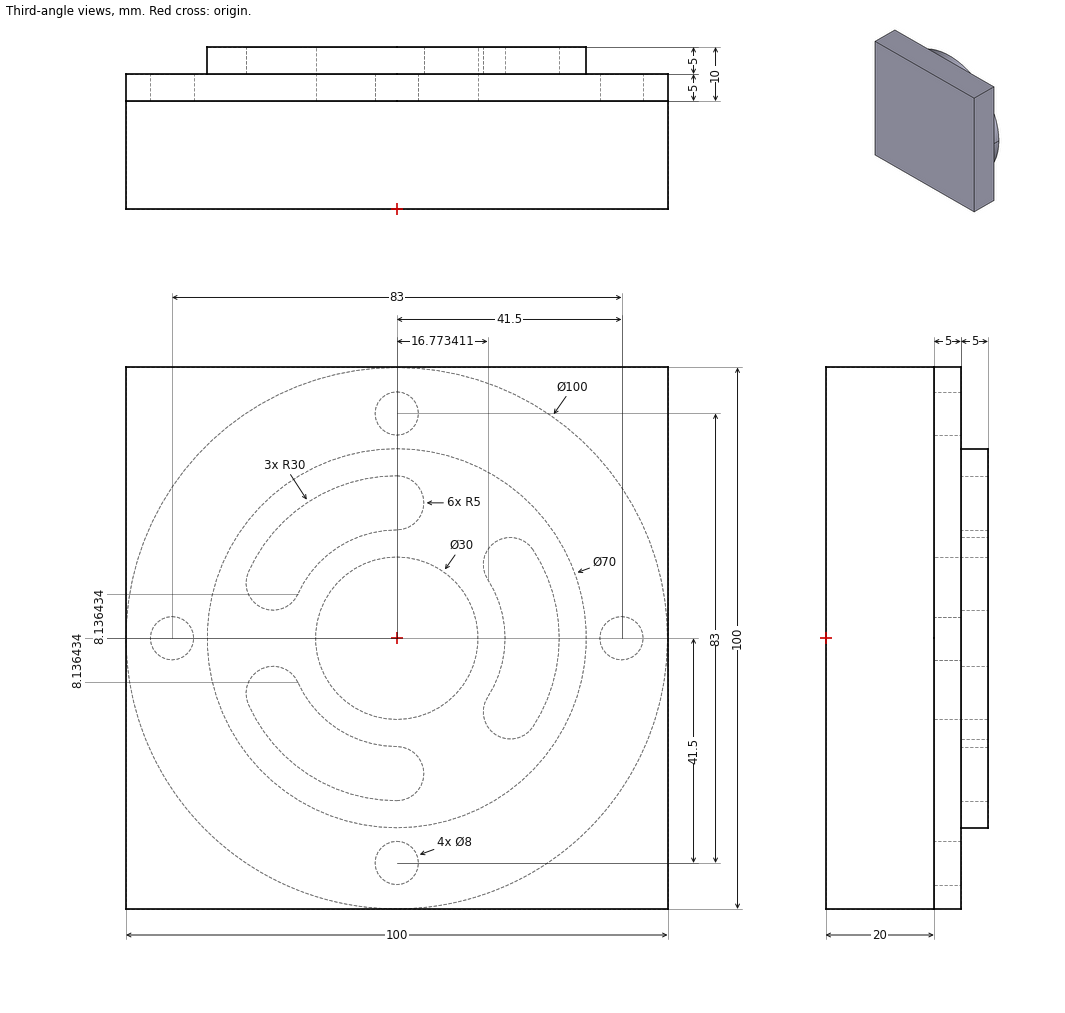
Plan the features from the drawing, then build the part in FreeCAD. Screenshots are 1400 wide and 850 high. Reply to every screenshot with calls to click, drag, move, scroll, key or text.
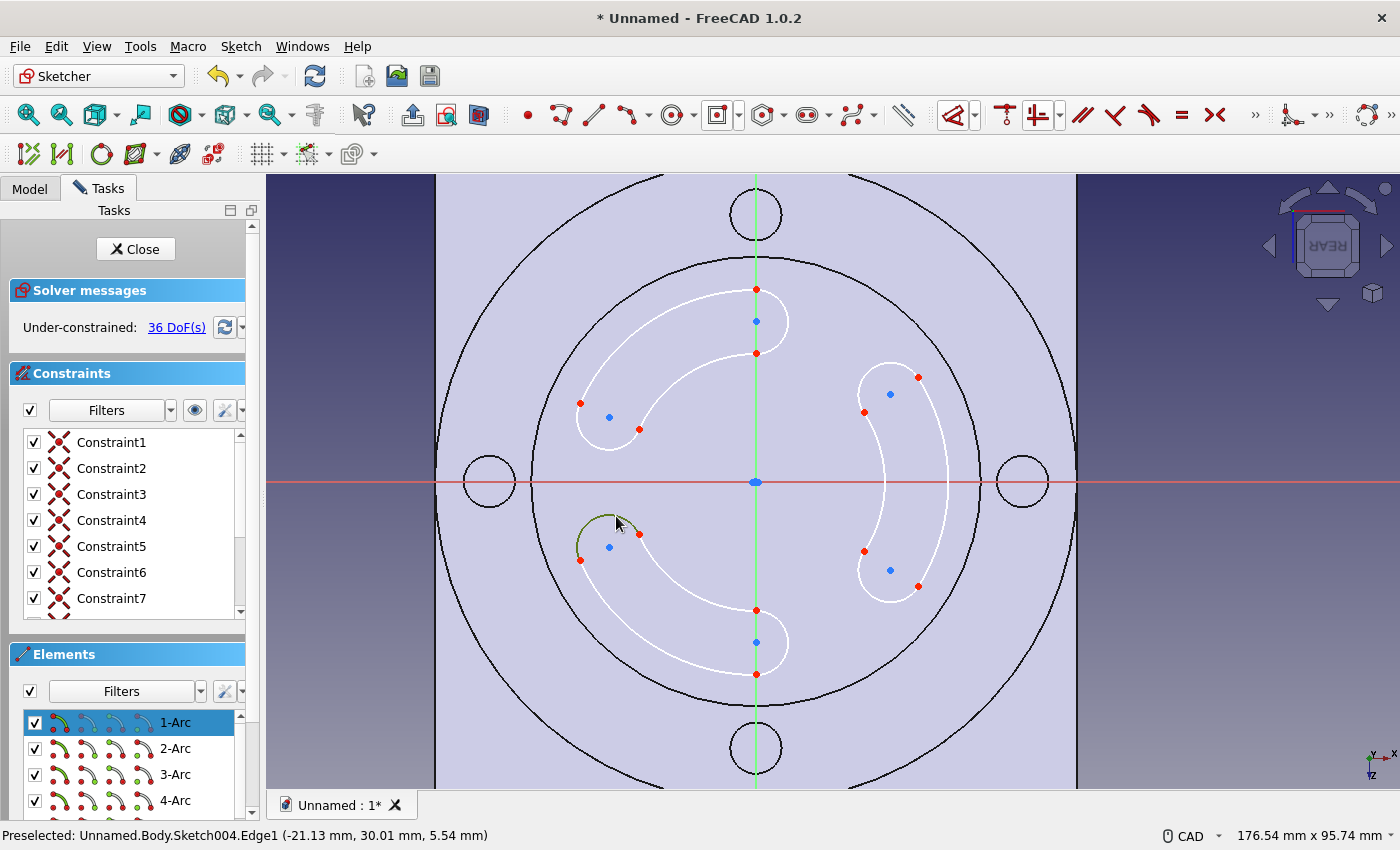
click(617, 616)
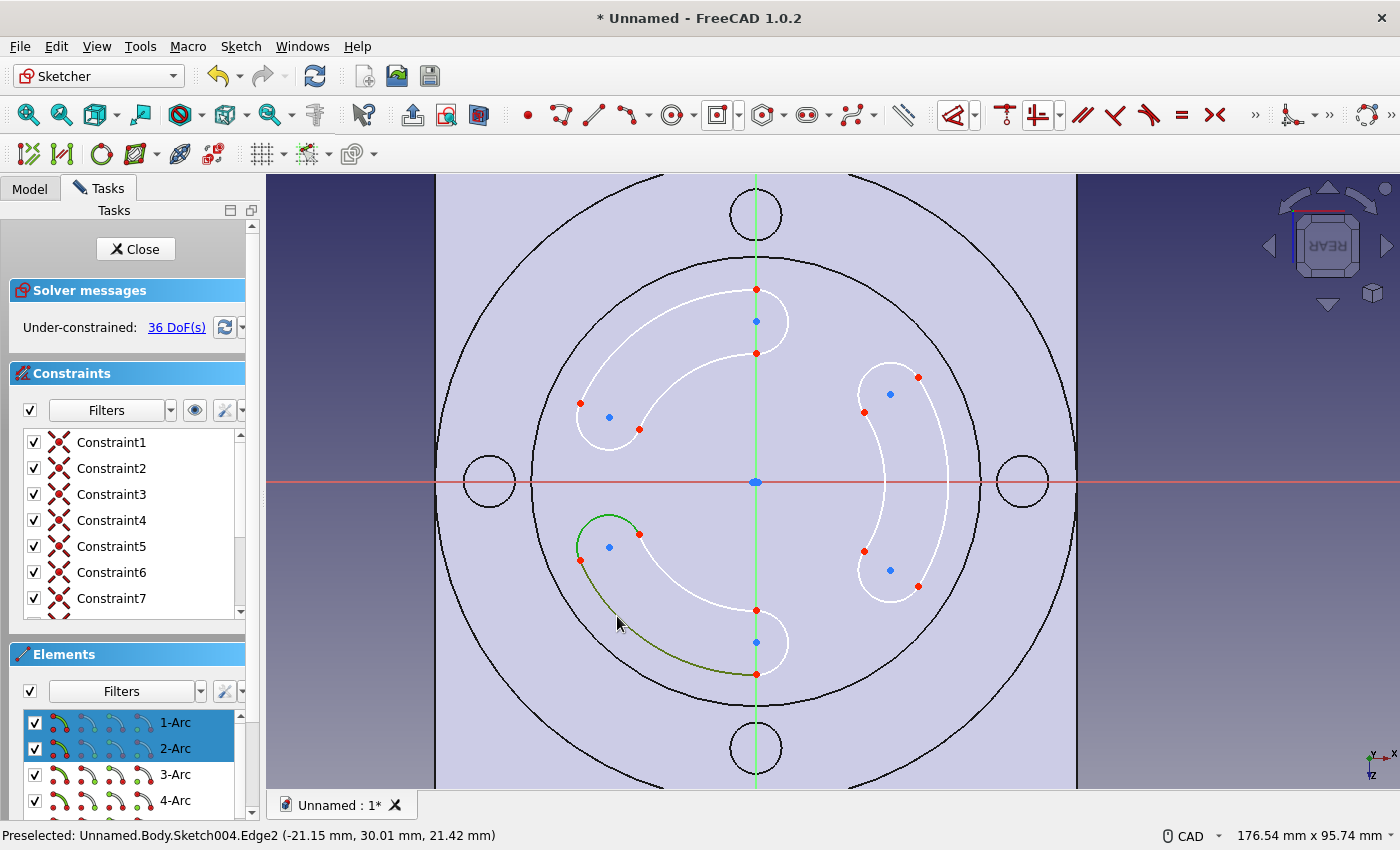
click(1149, 116)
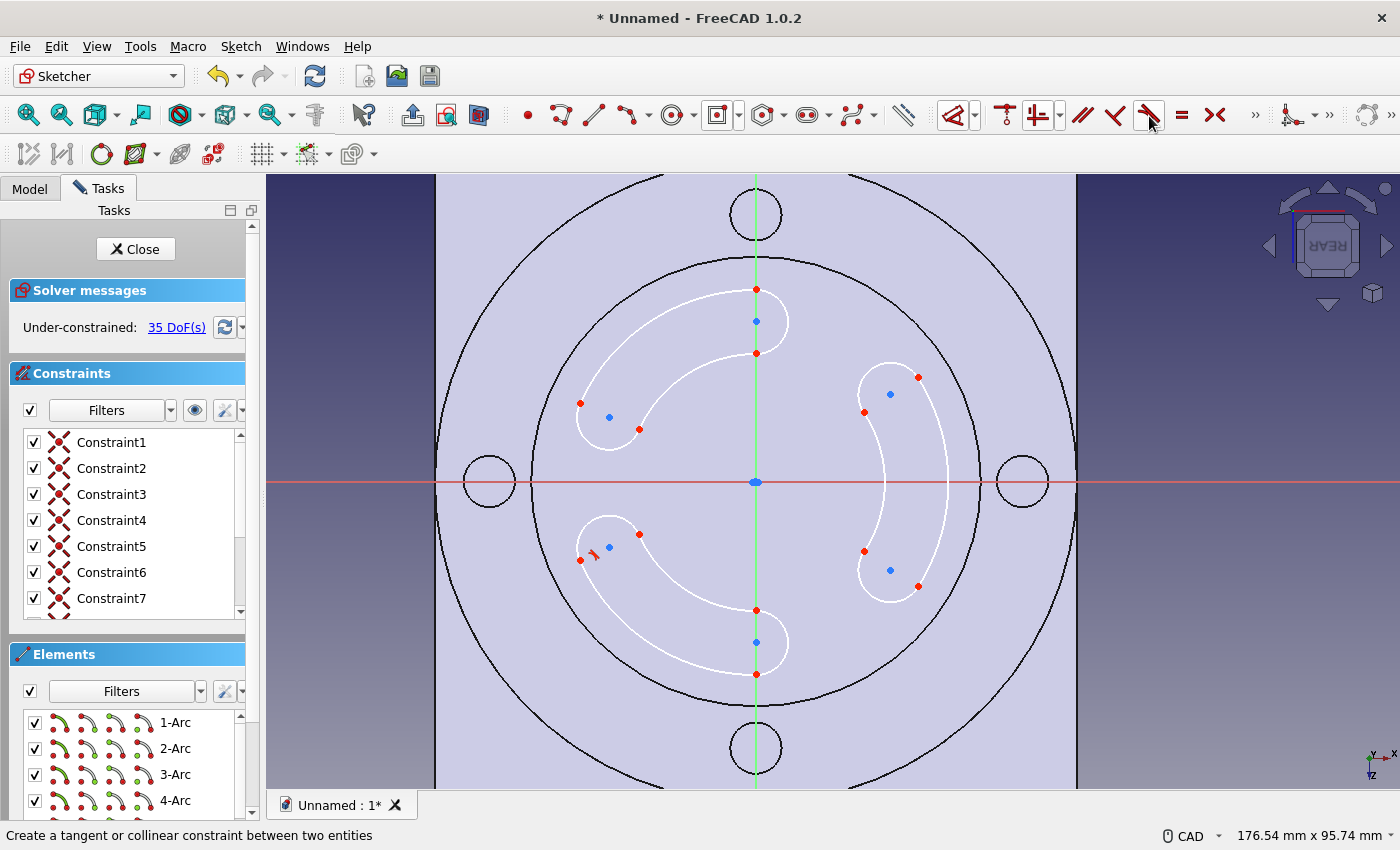
click(616, 516)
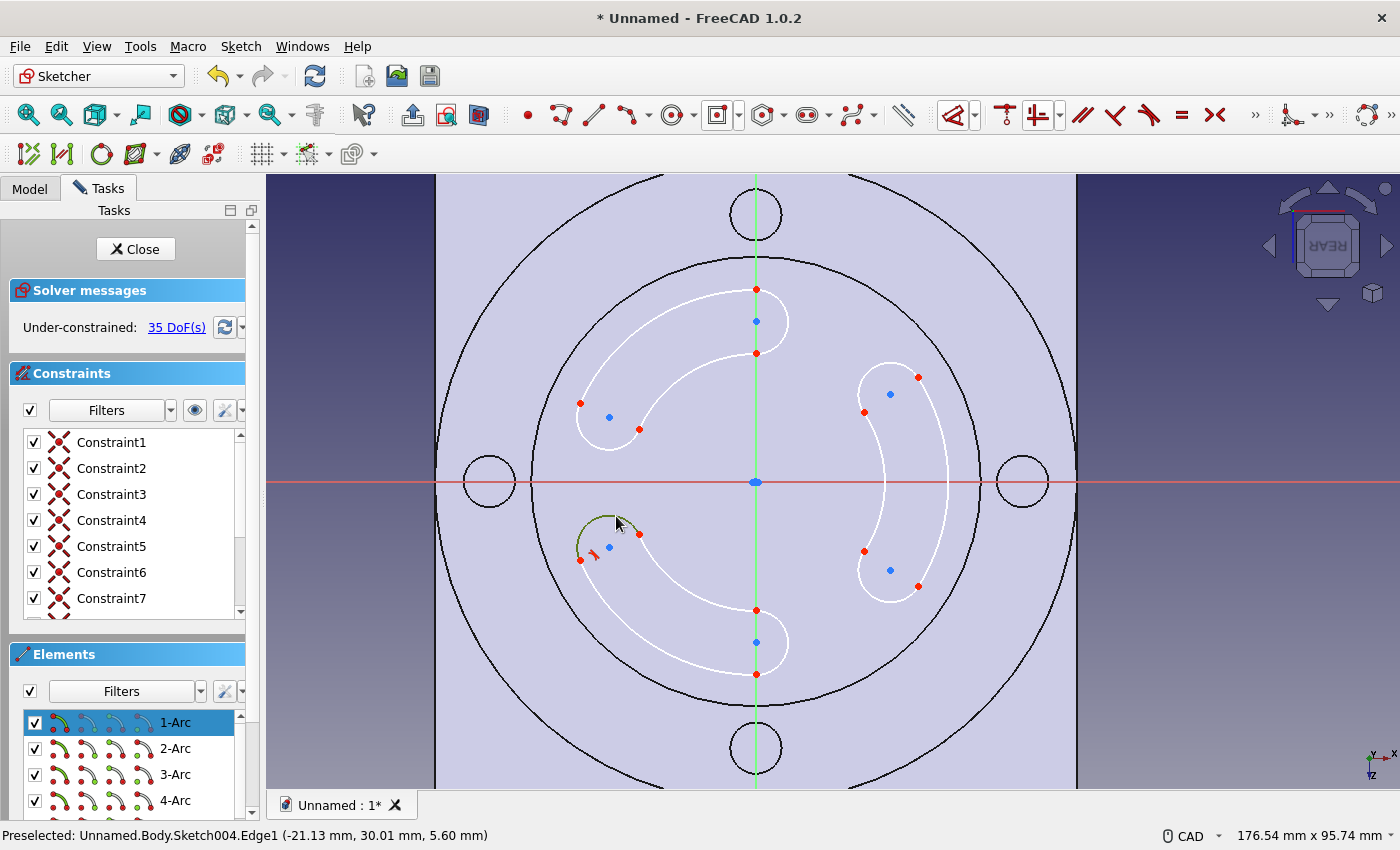
click(664, 571)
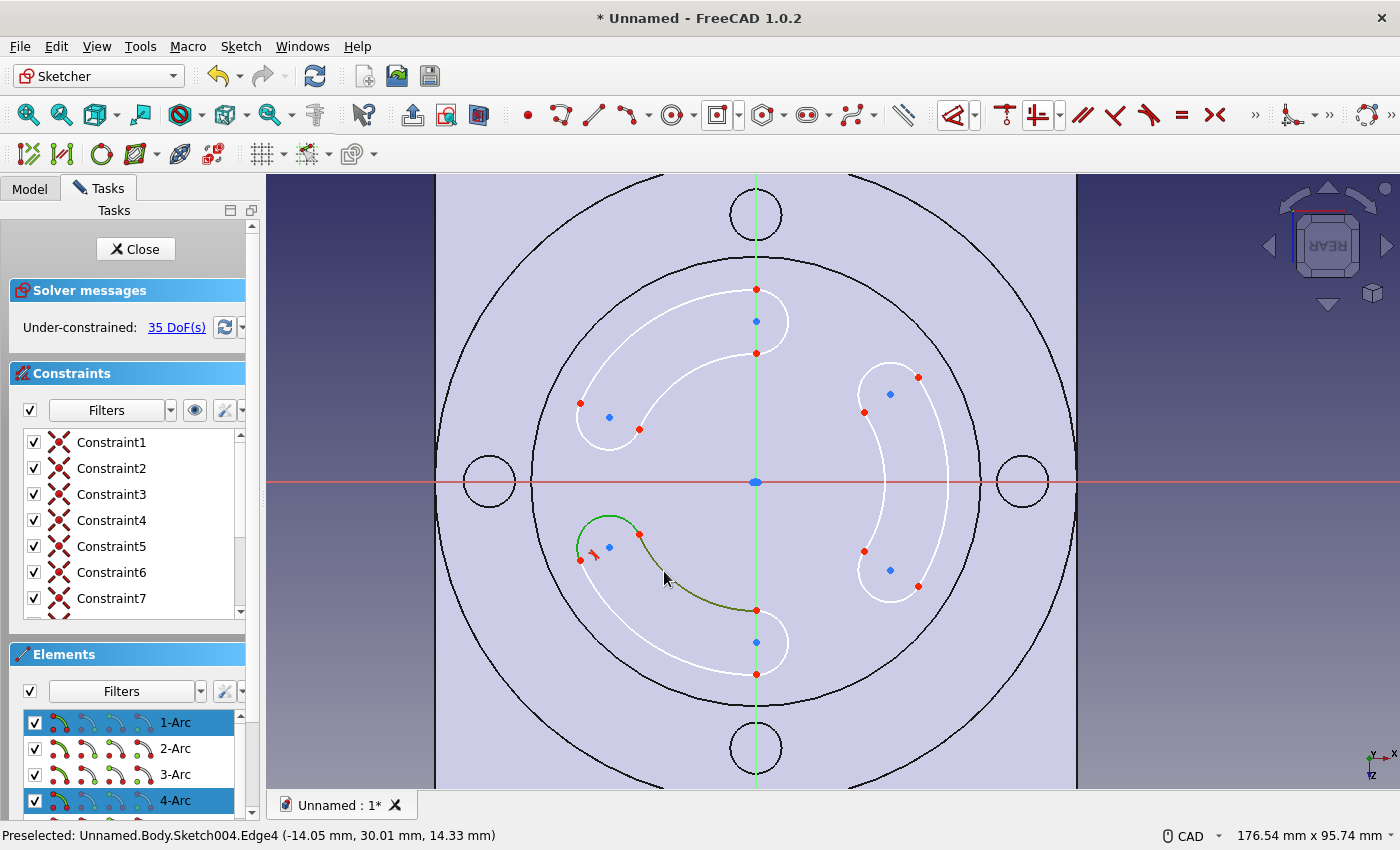
click(1149, 116)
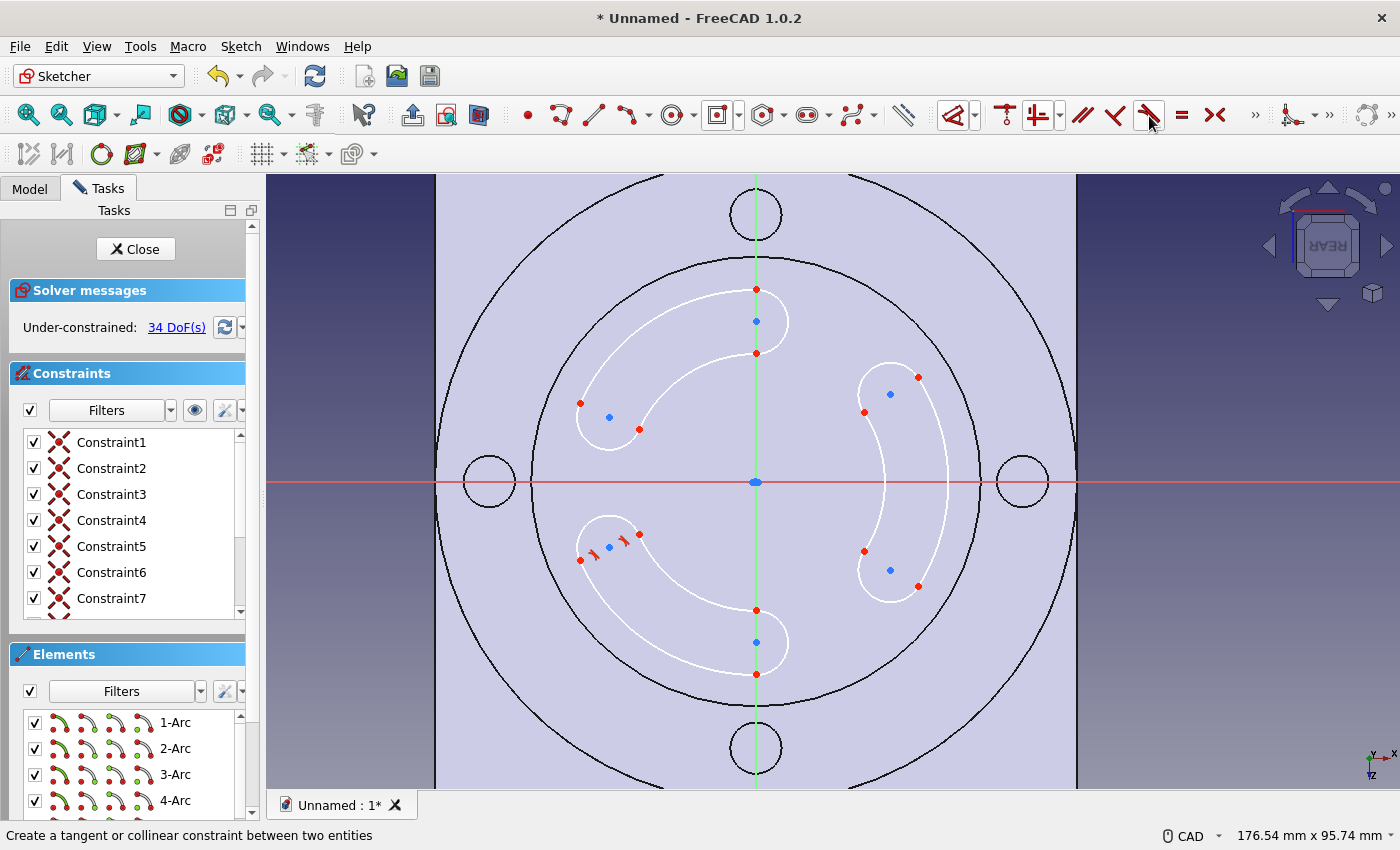
click(617, 616)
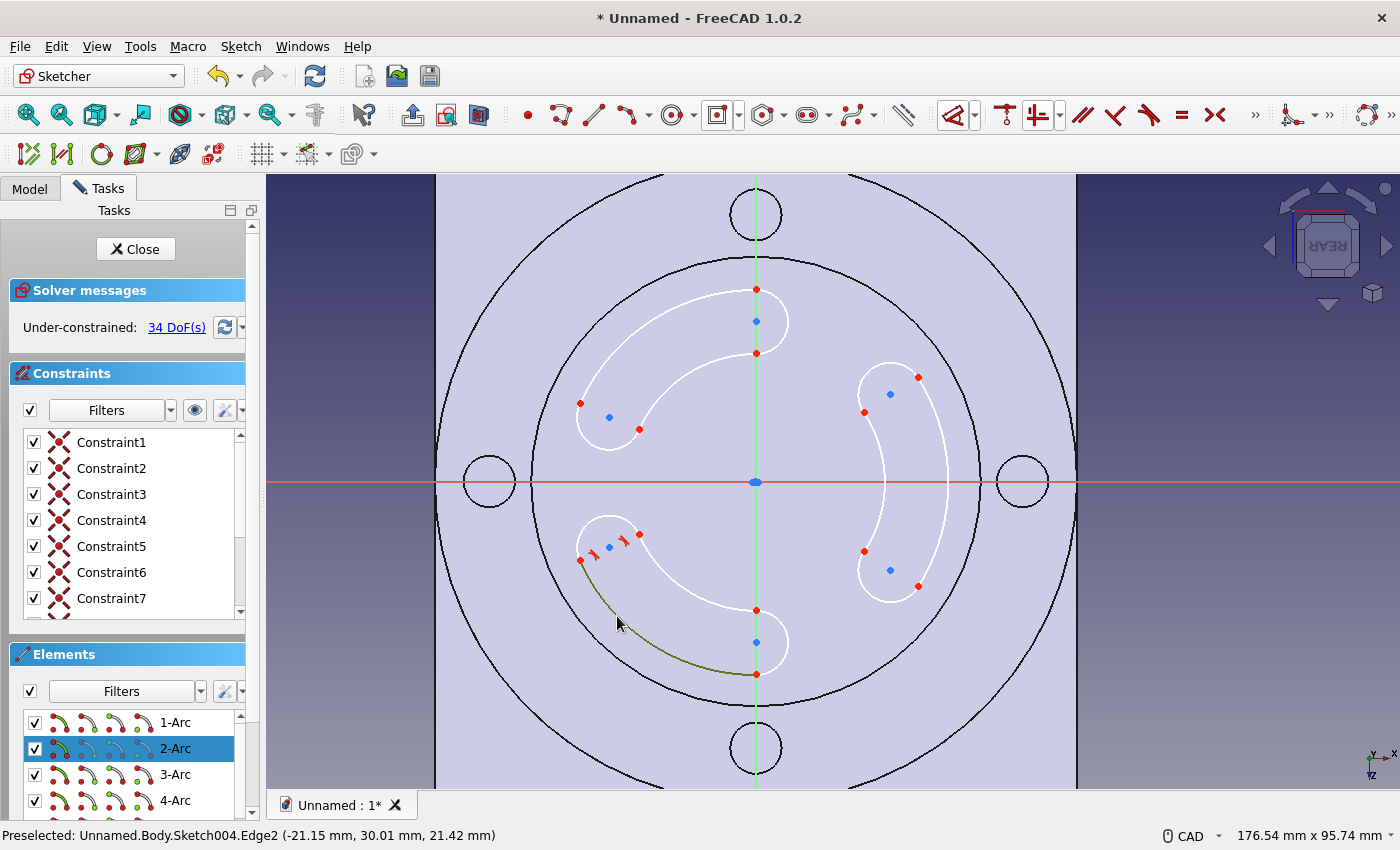
click(782, 662)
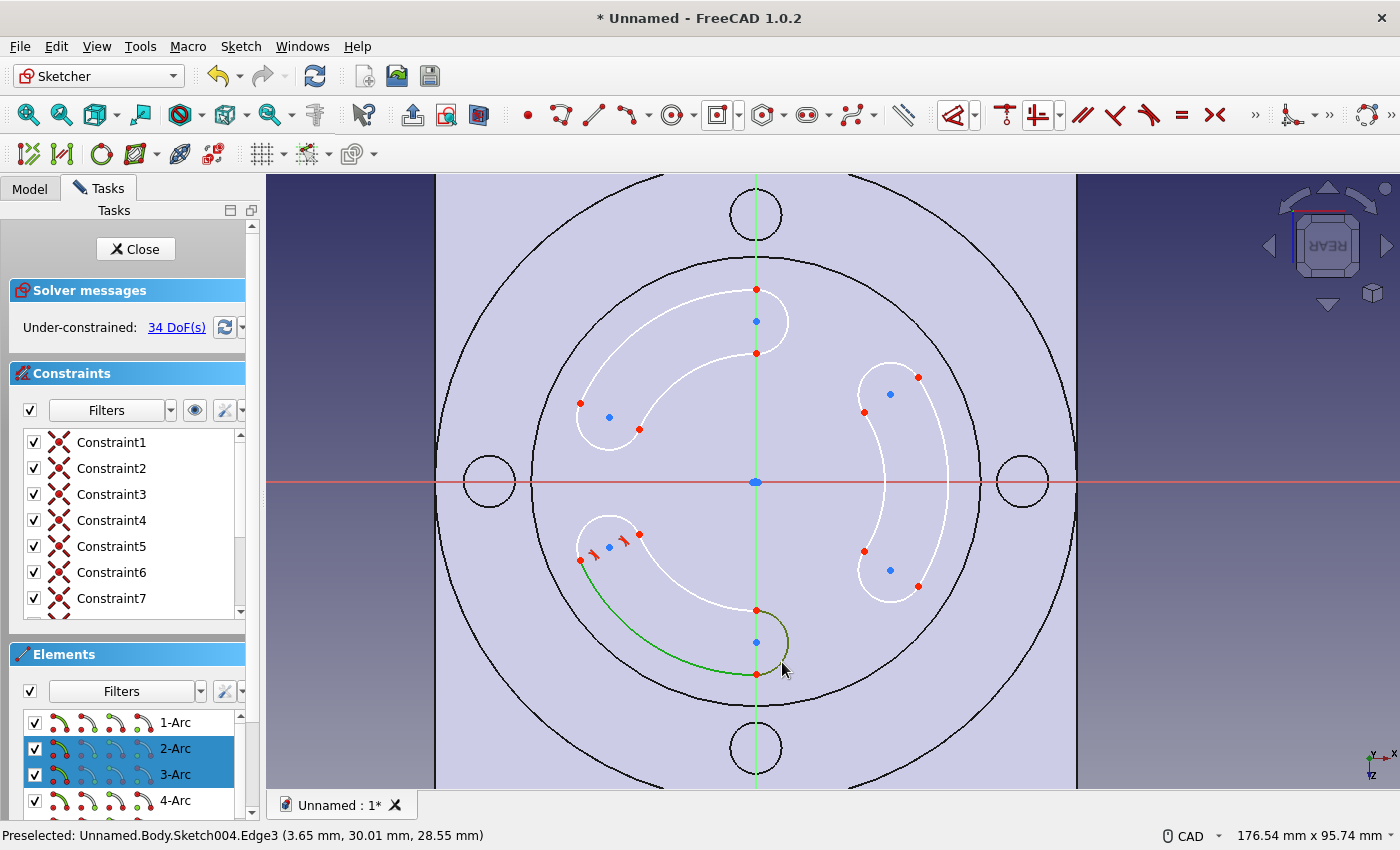
click(1149, 116)